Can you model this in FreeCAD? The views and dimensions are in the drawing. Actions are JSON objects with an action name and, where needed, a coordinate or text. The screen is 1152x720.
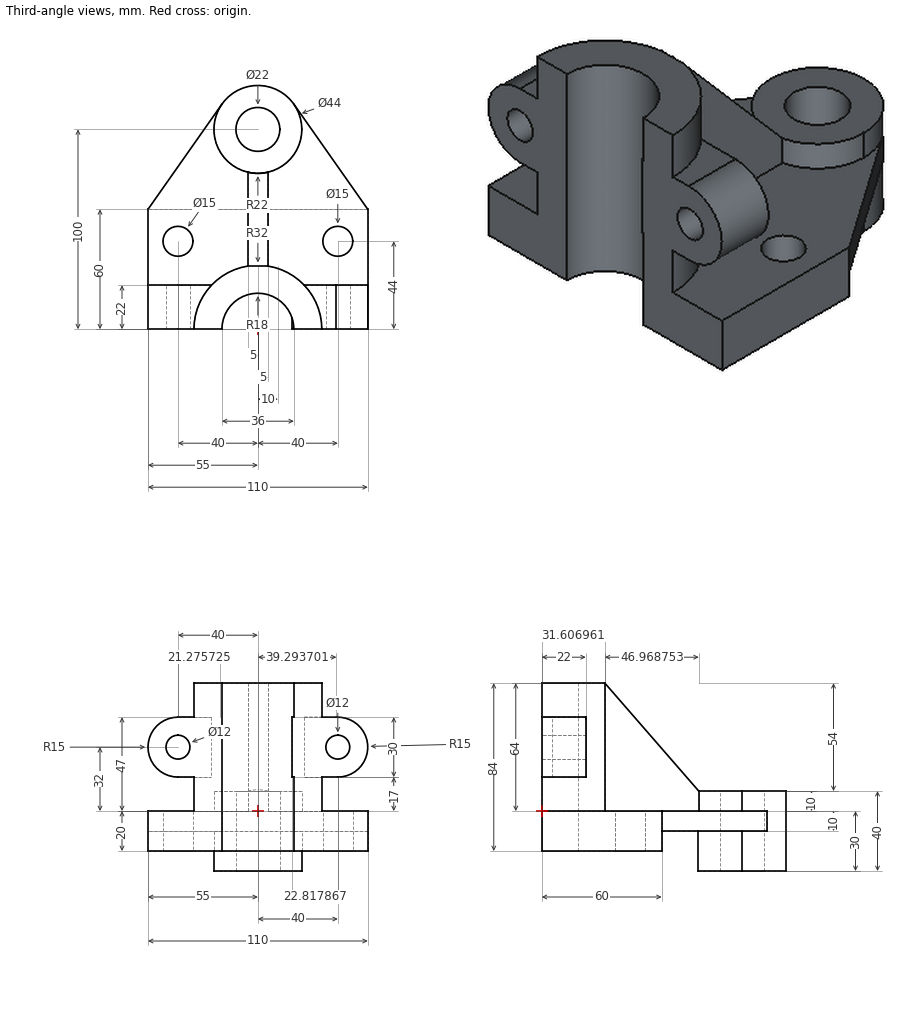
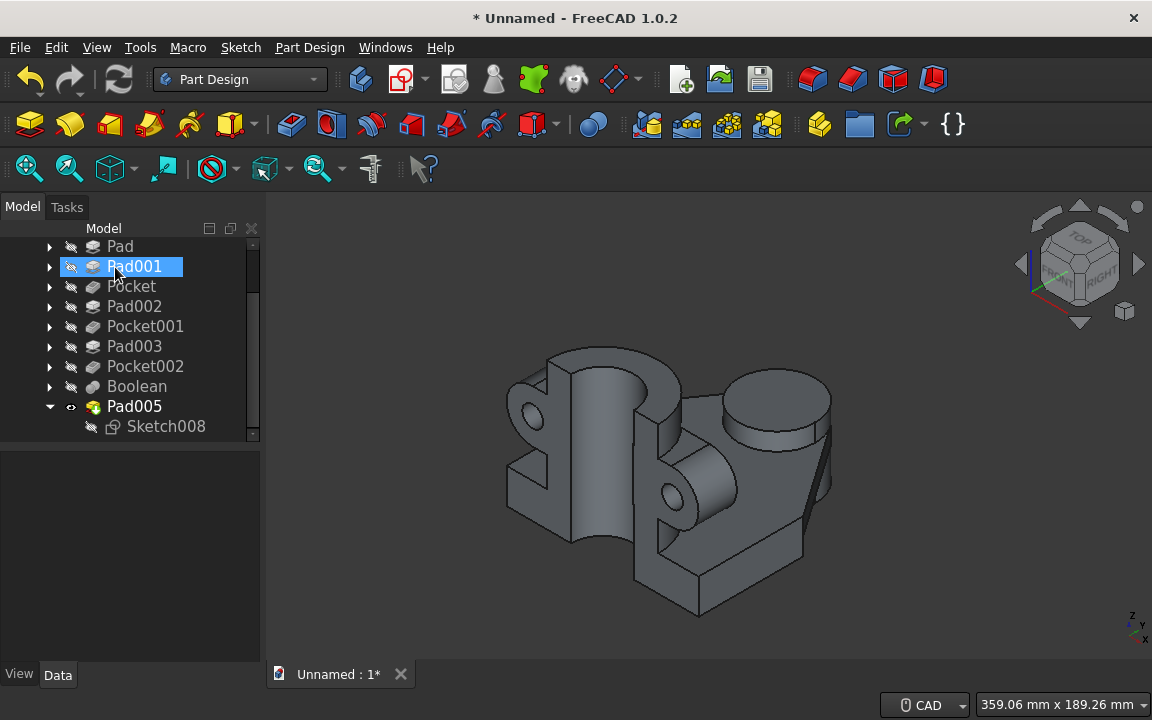
{"action": "left_click", "coordinate": [777, 399]}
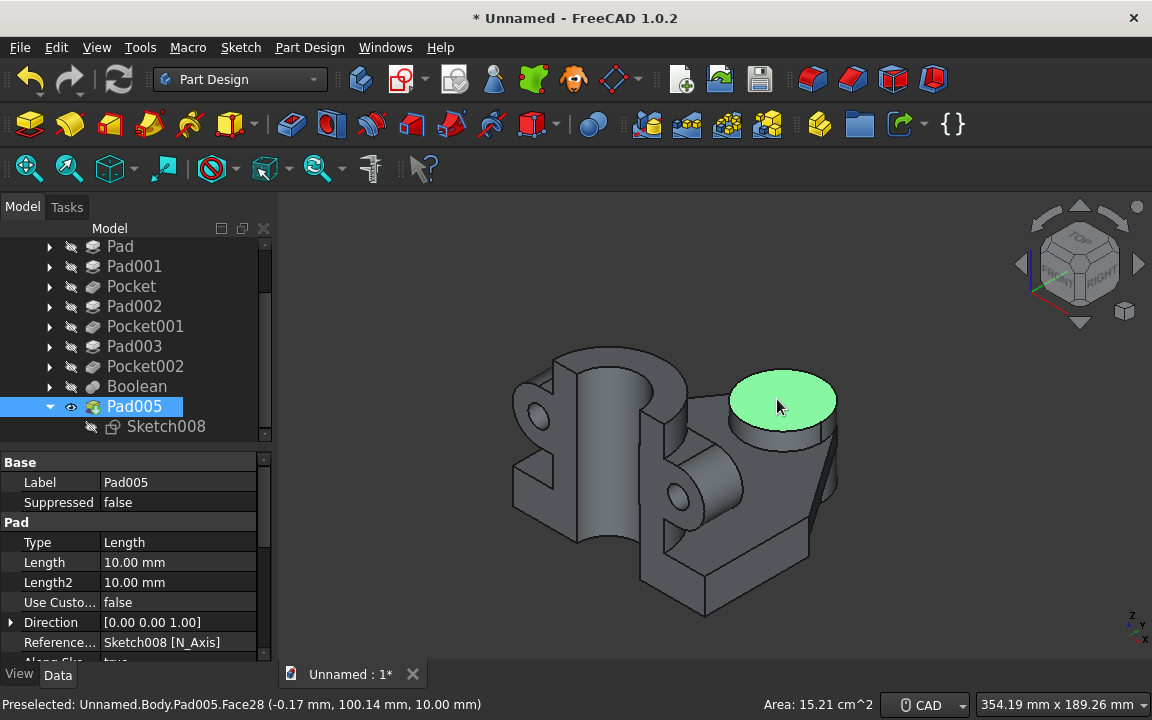
{"action": "left_click", "coordinate": [402, 80]}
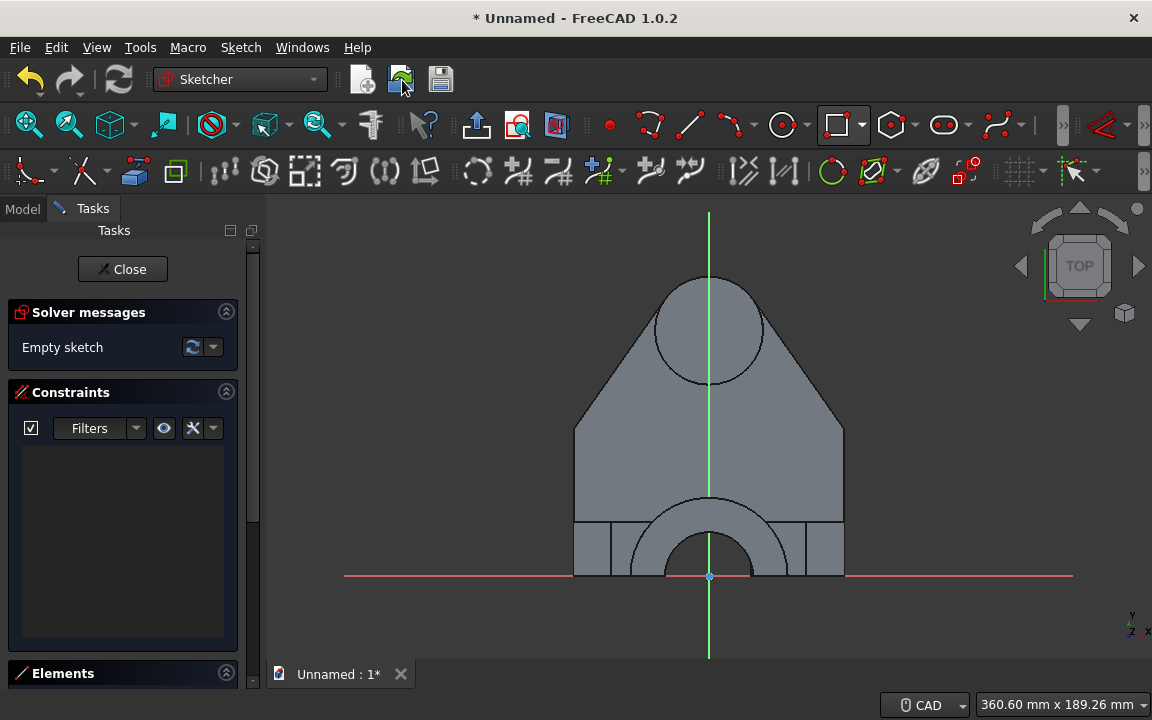
{"action": "left_click", "coordinate": [558, 126]}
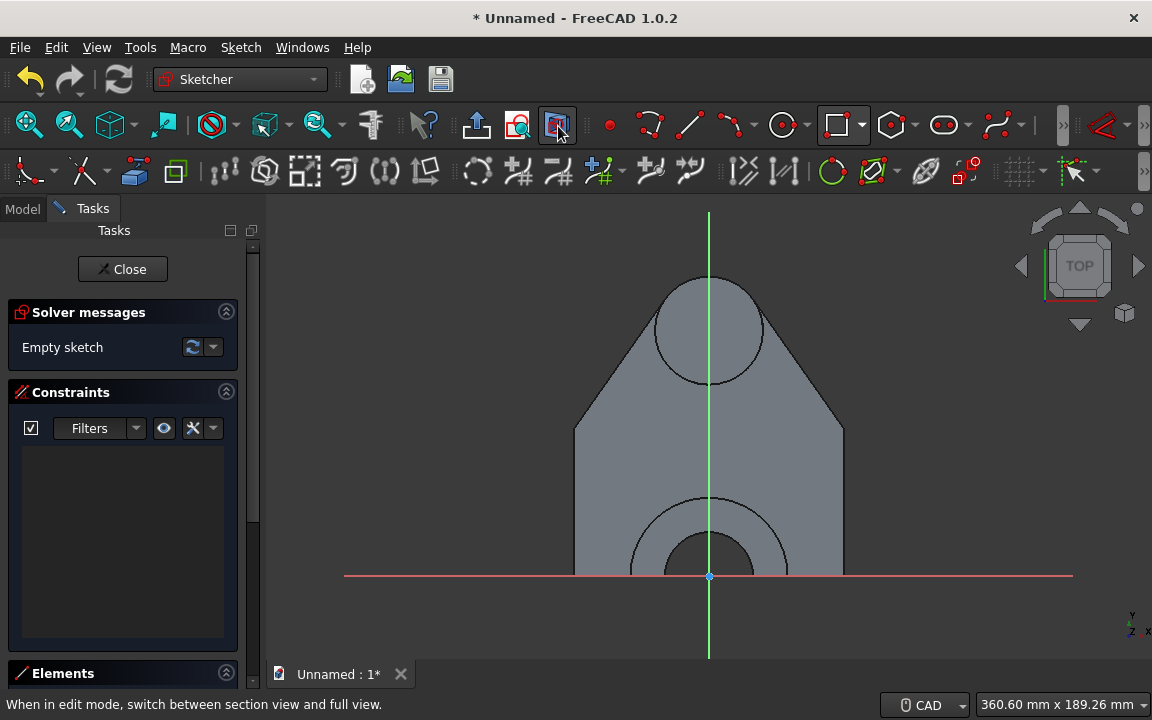
{"action": "scroll", "coordinate": [726, 306], "scroll_direction": "up", "scroll_amount": 8}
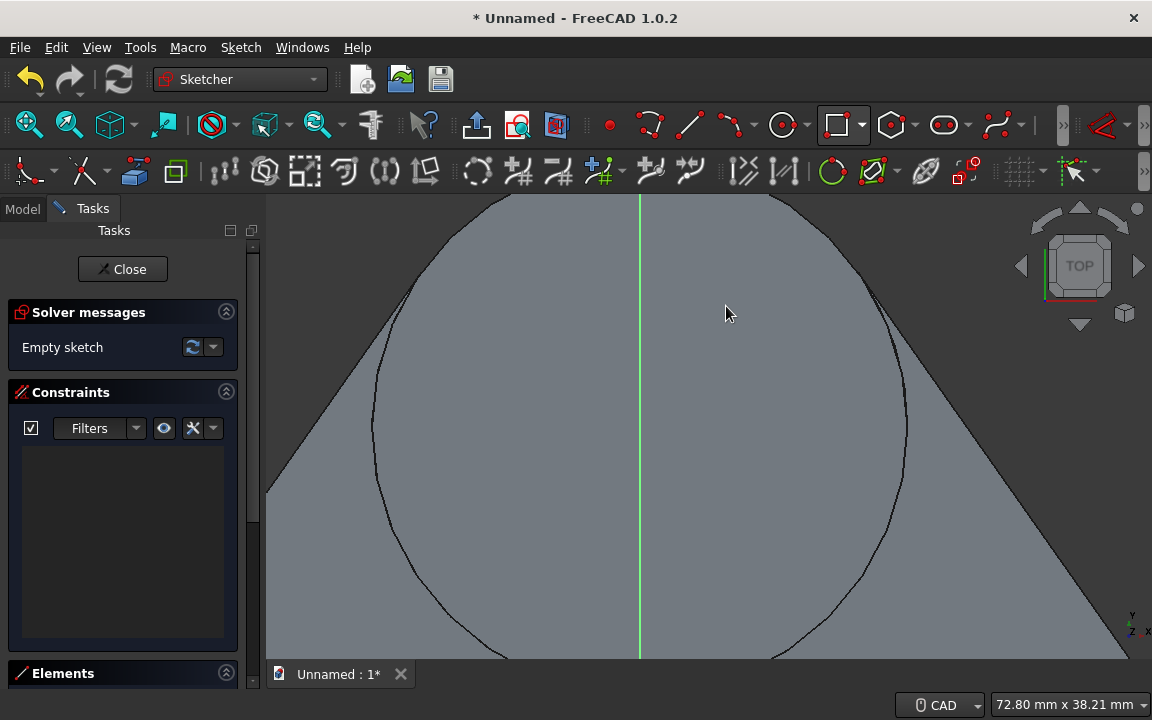
{"action": "left_click", "coordinate": [784, 126]}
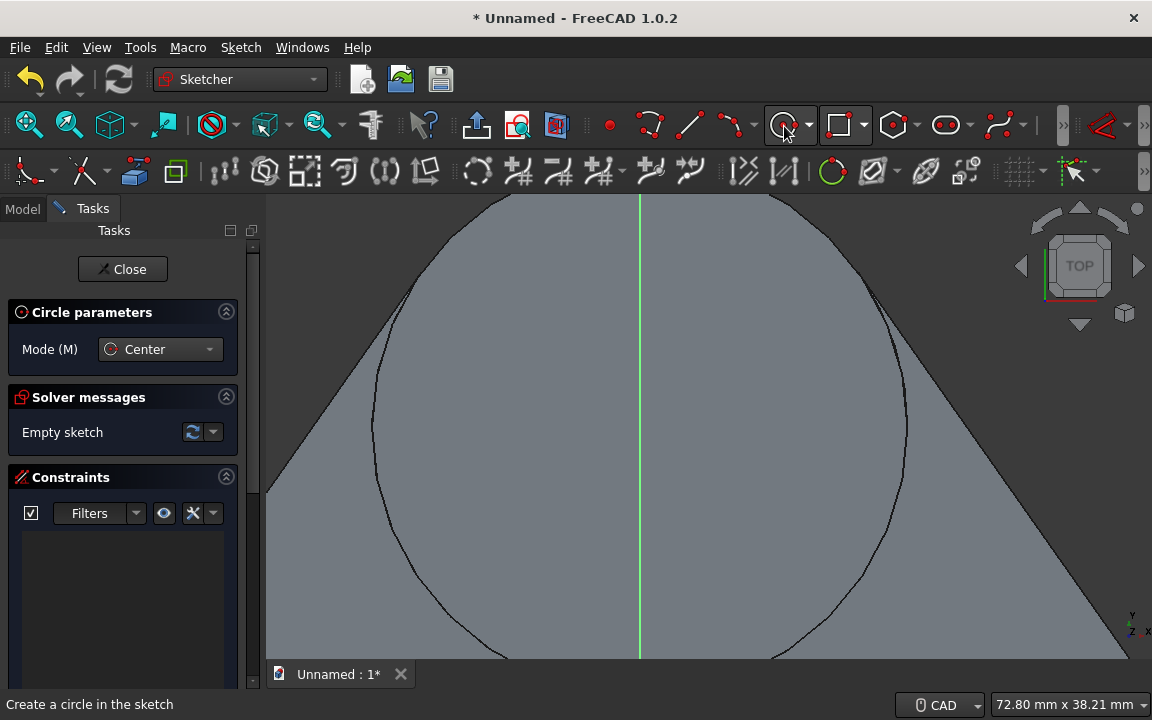
{"action": "left_click", "coordinate": [640, 427]}
{"action": "left_click", "coordinate": [734, 333]}
{"action": "key", "text": "Escape"}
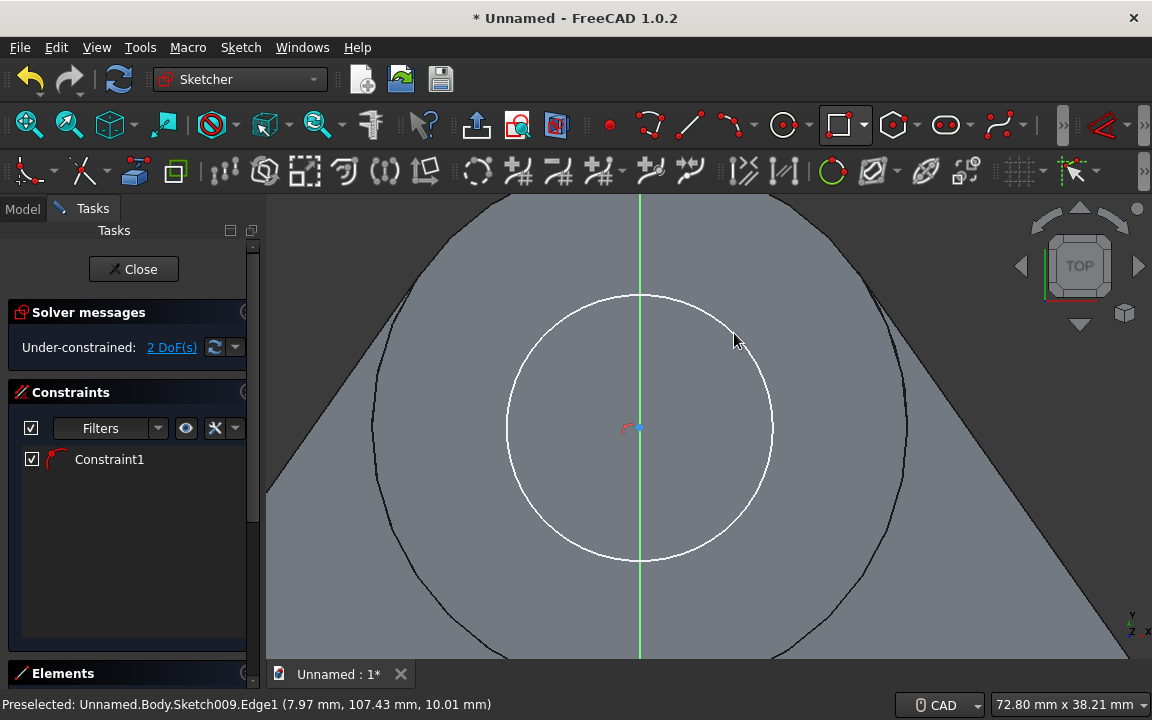
{"action": "left_click", "coordinate": [1102, 126]}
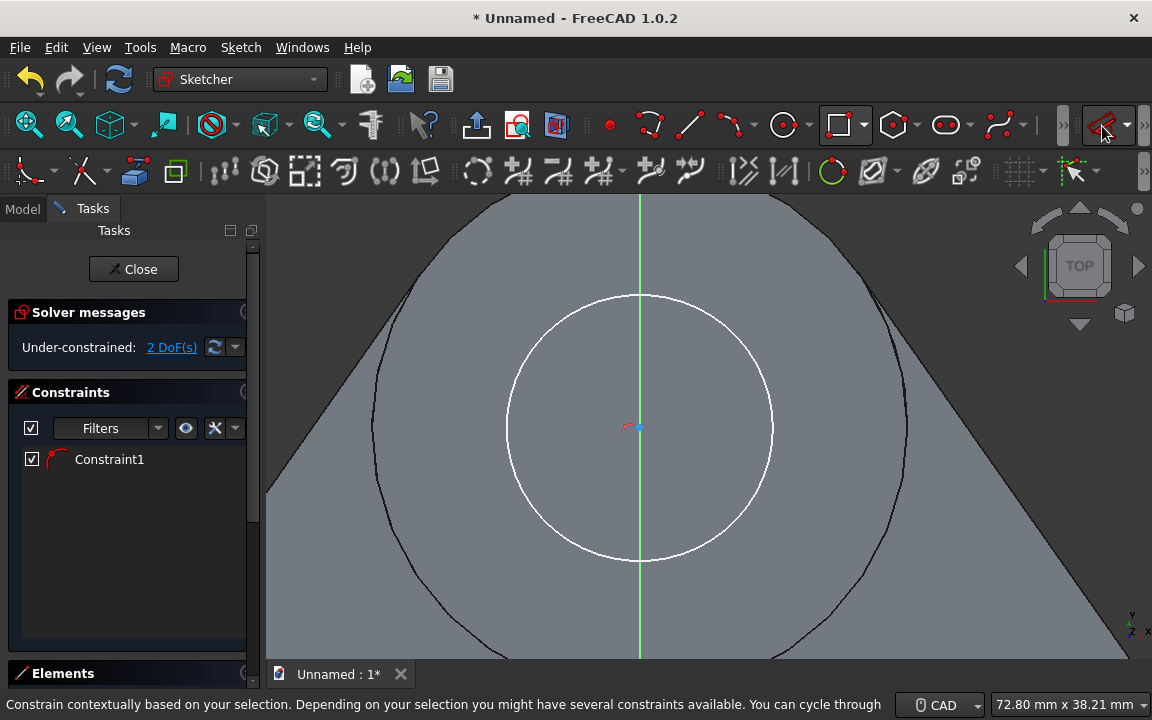
{"action": "left_click", "coordinate": [734, 334]}
{"action": "left_click", "coordinate": [757, 311]}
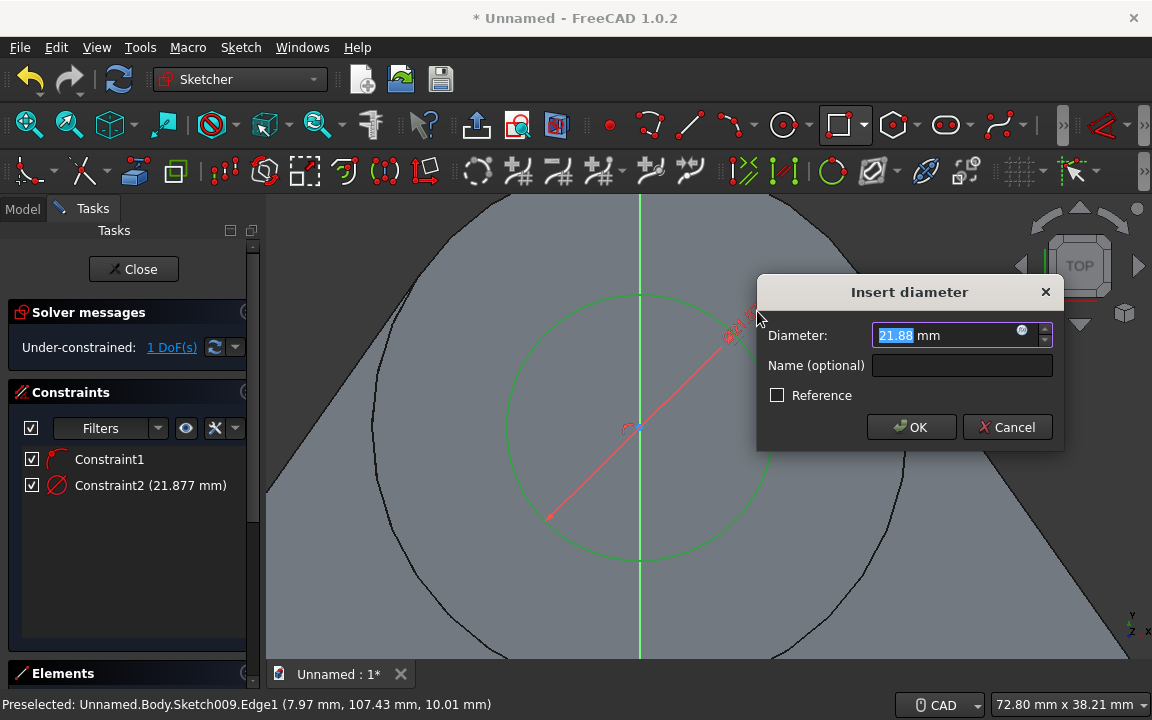
{"action": "type", "text": "22"}
{"action": "key", "text": "Return"}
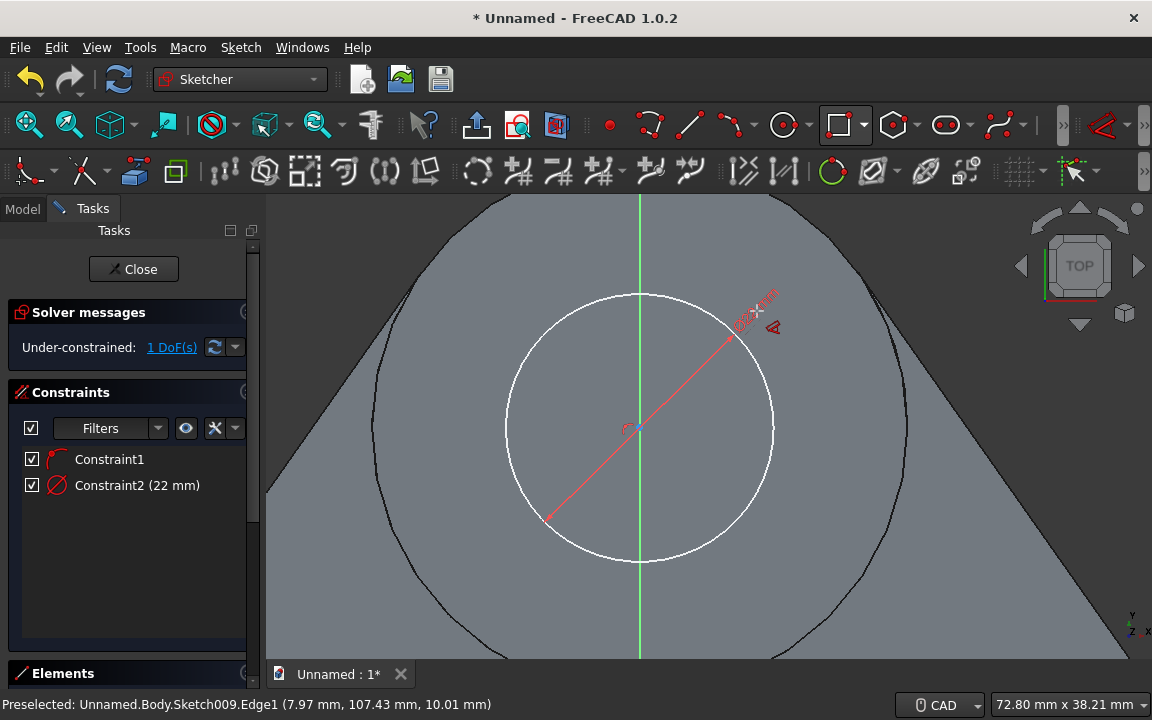
{"action": "left_click", "coordinate": [640, 428]}
{"action": "left_click", "coordinate": [674, 530]}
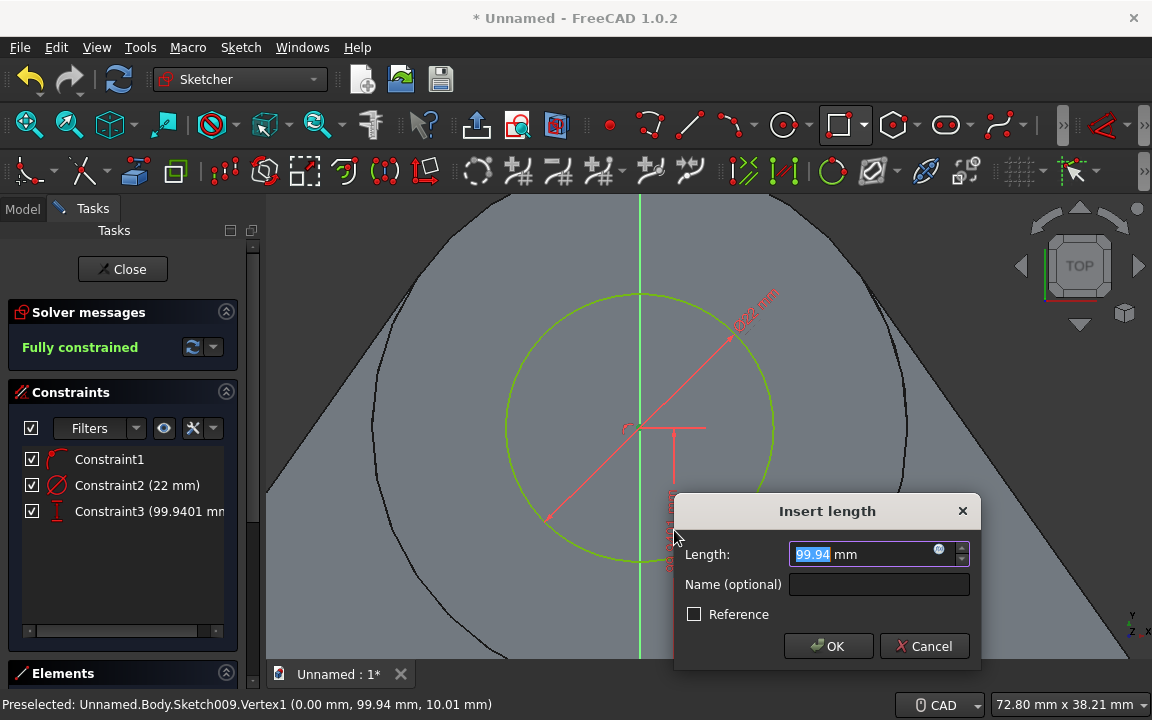
{"action": "type", "text": "100"}
{"action": "key", "text": "Return"}
{"action": "key", "text": "Escape"}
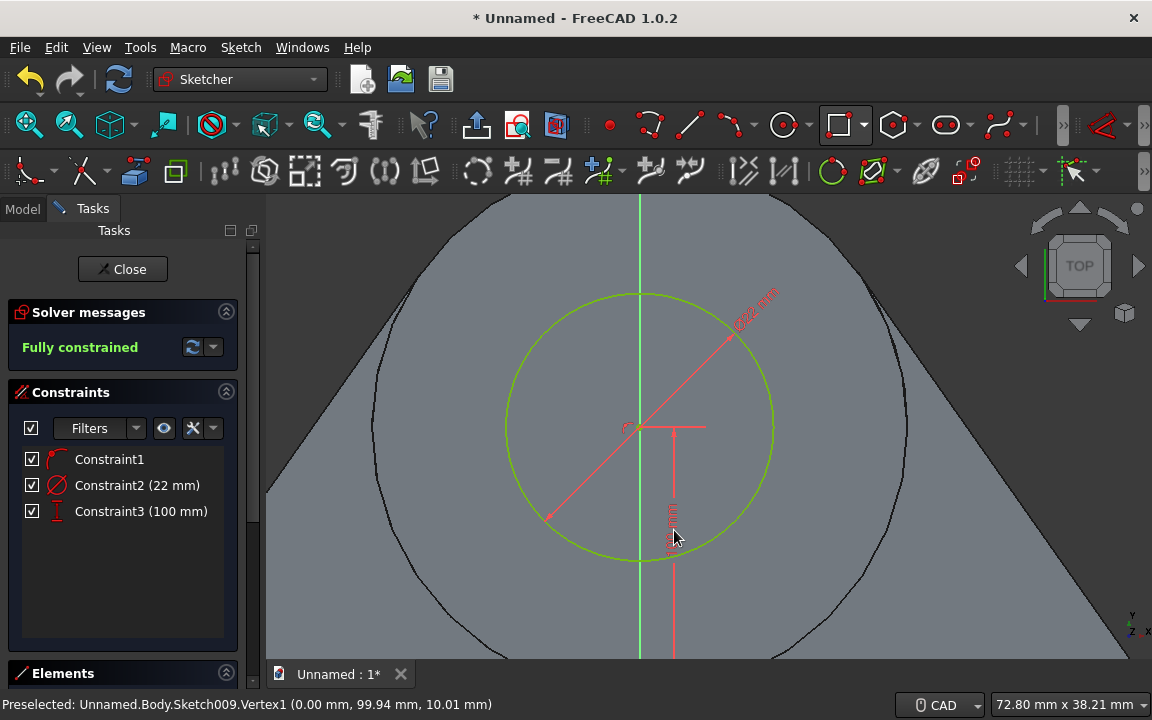
{"action": "left_click", "coordinate": [123, 269]}